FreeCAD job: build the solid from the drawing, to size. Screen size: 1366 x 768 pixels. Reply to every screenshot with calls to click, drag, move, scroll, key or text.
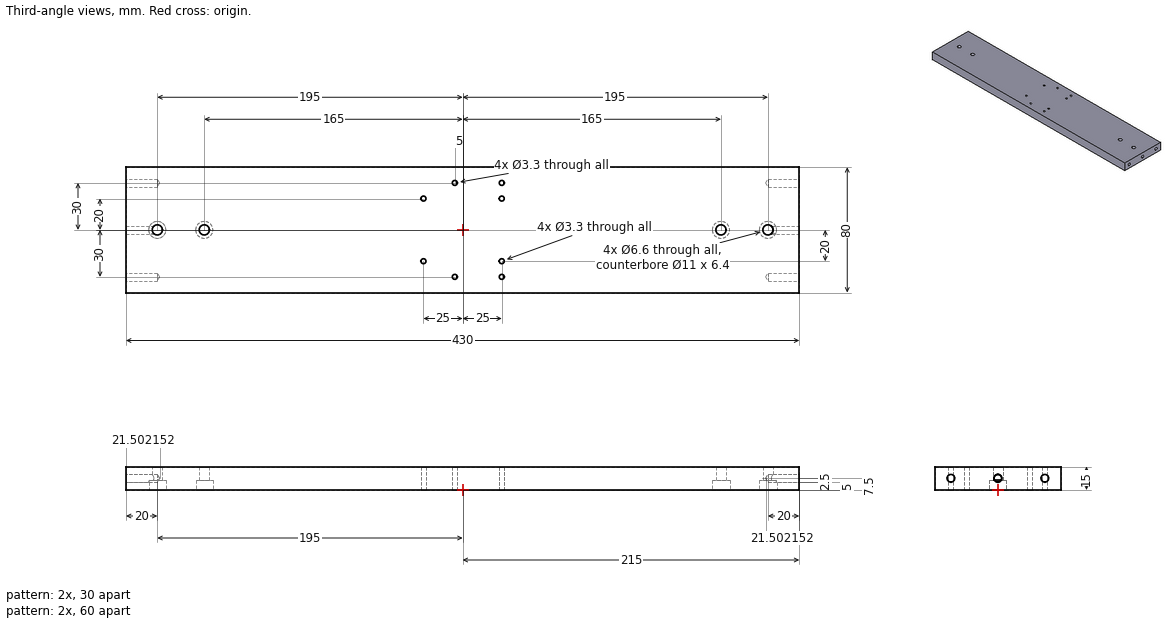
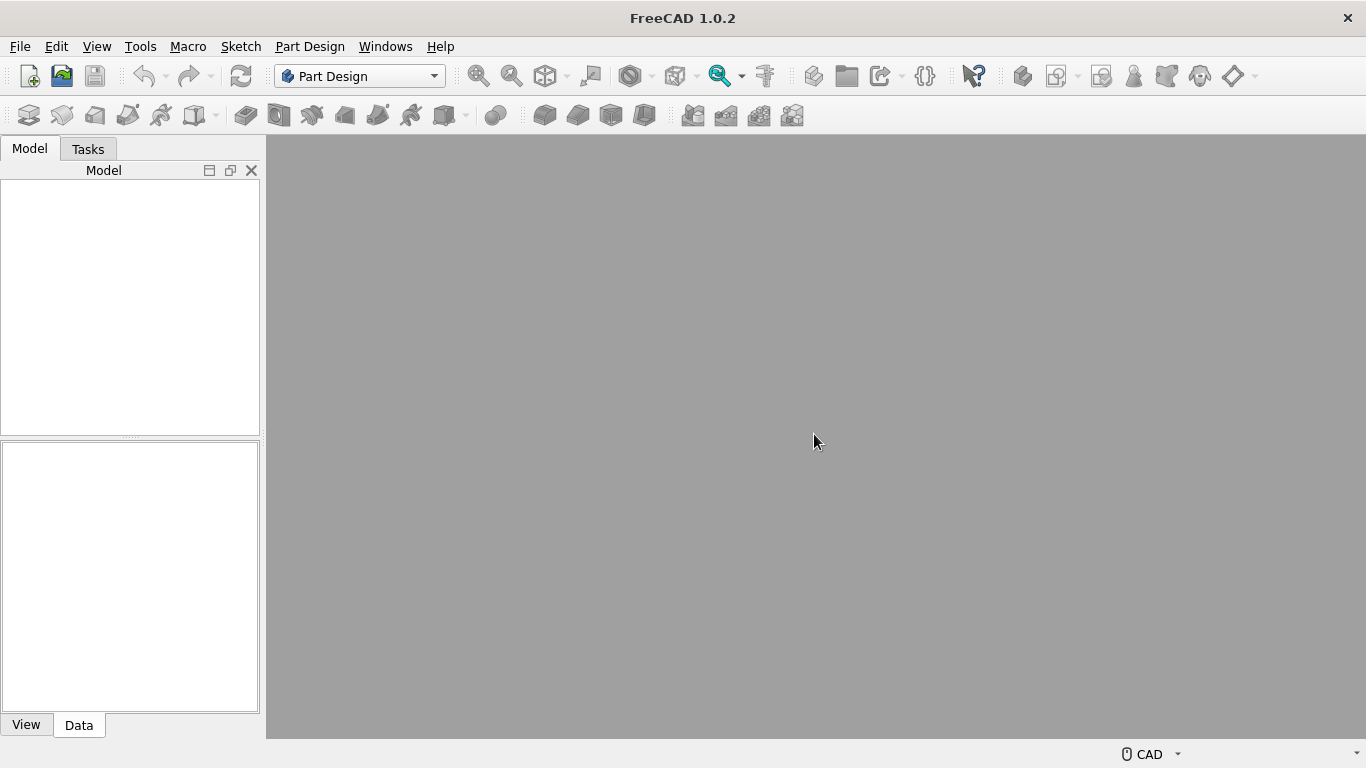
click(29, 76)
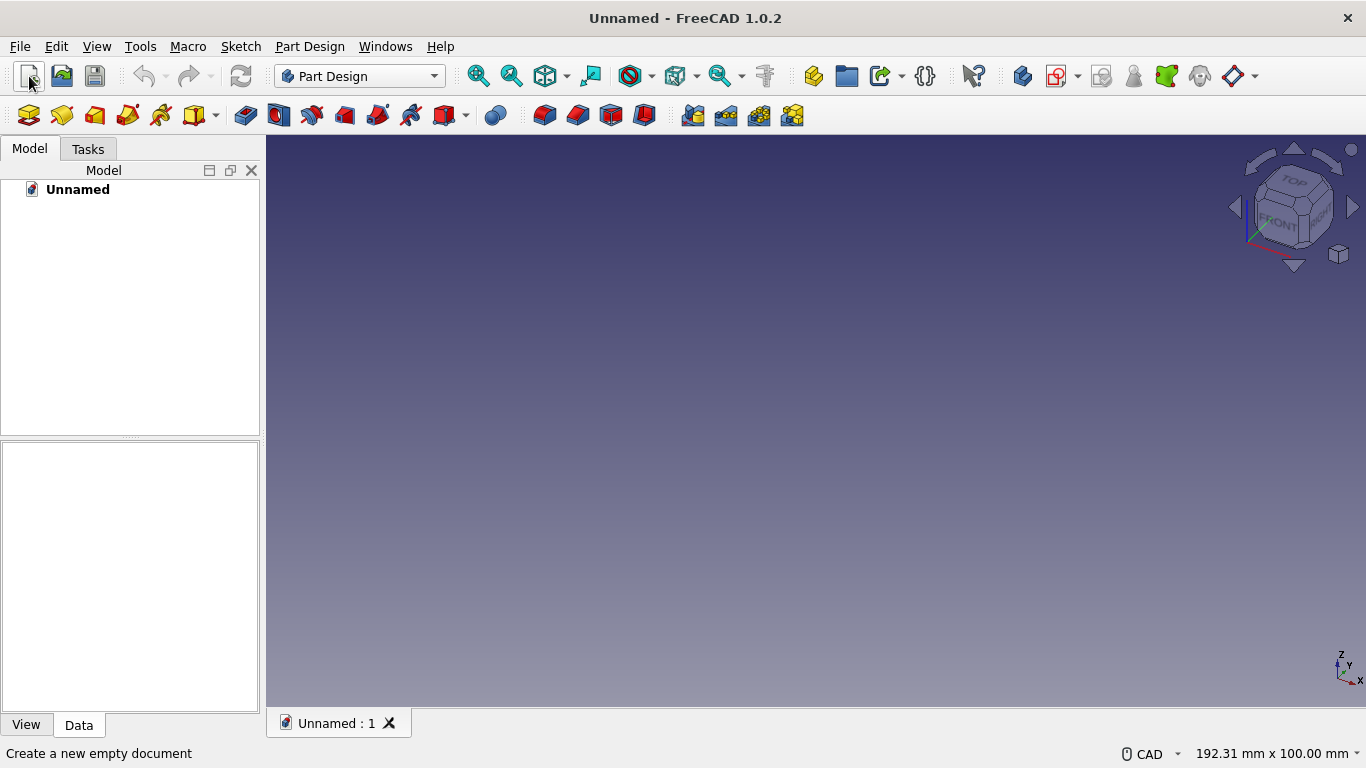
click(1056, 76)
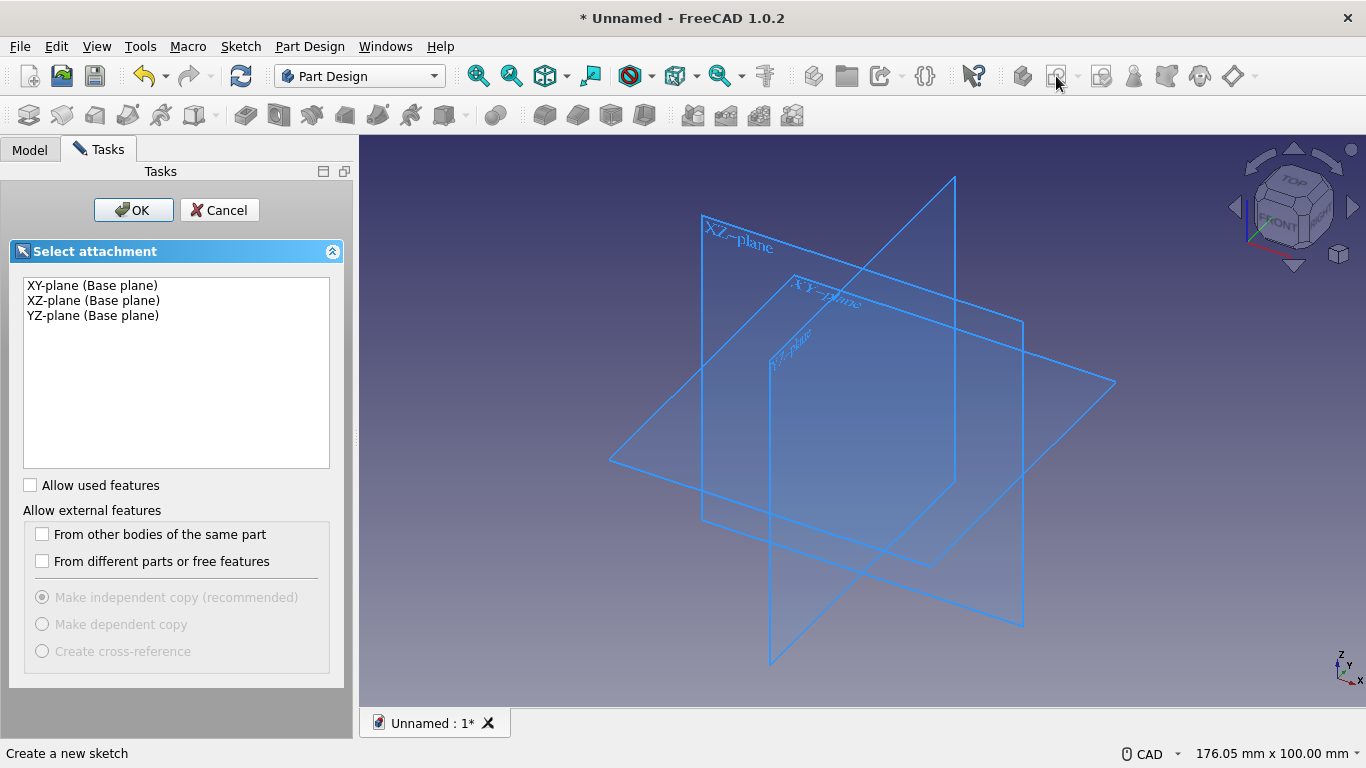
click(84, 286)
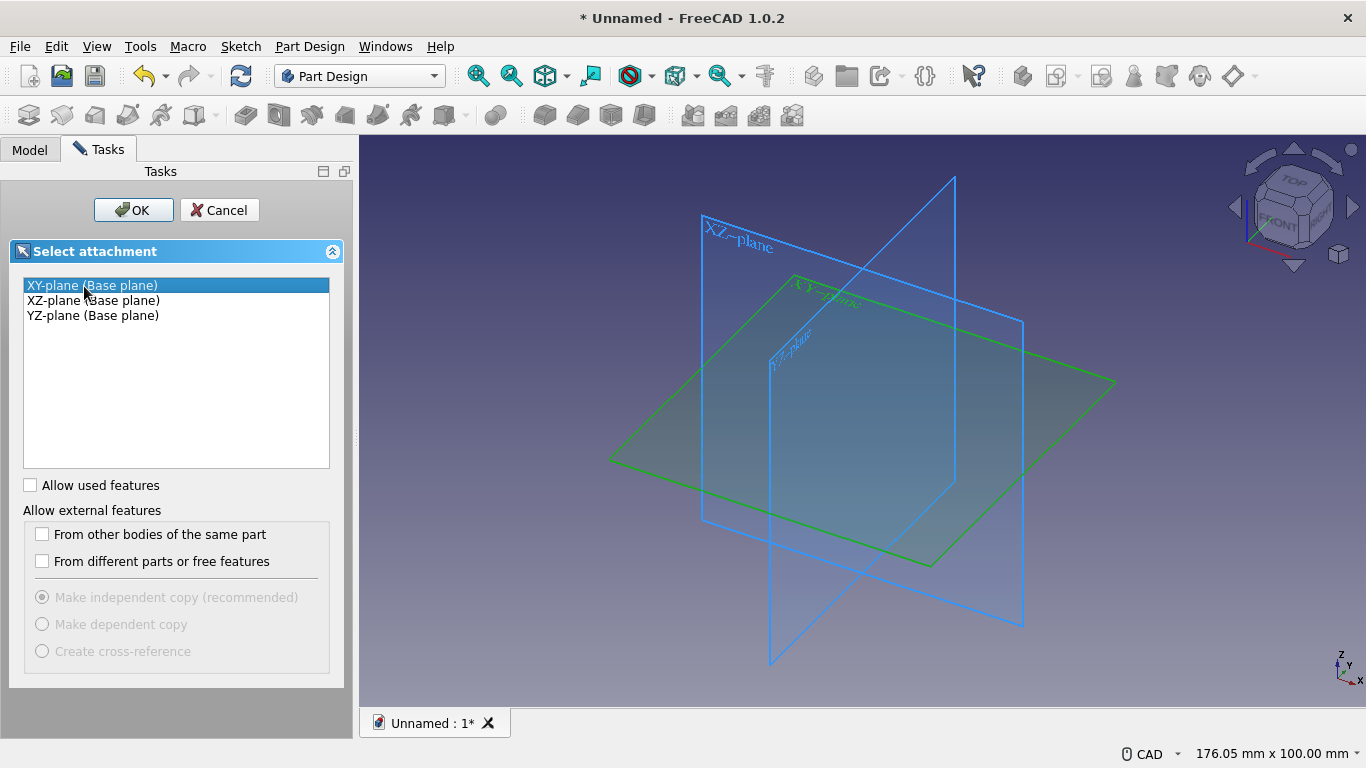
click(134, 210)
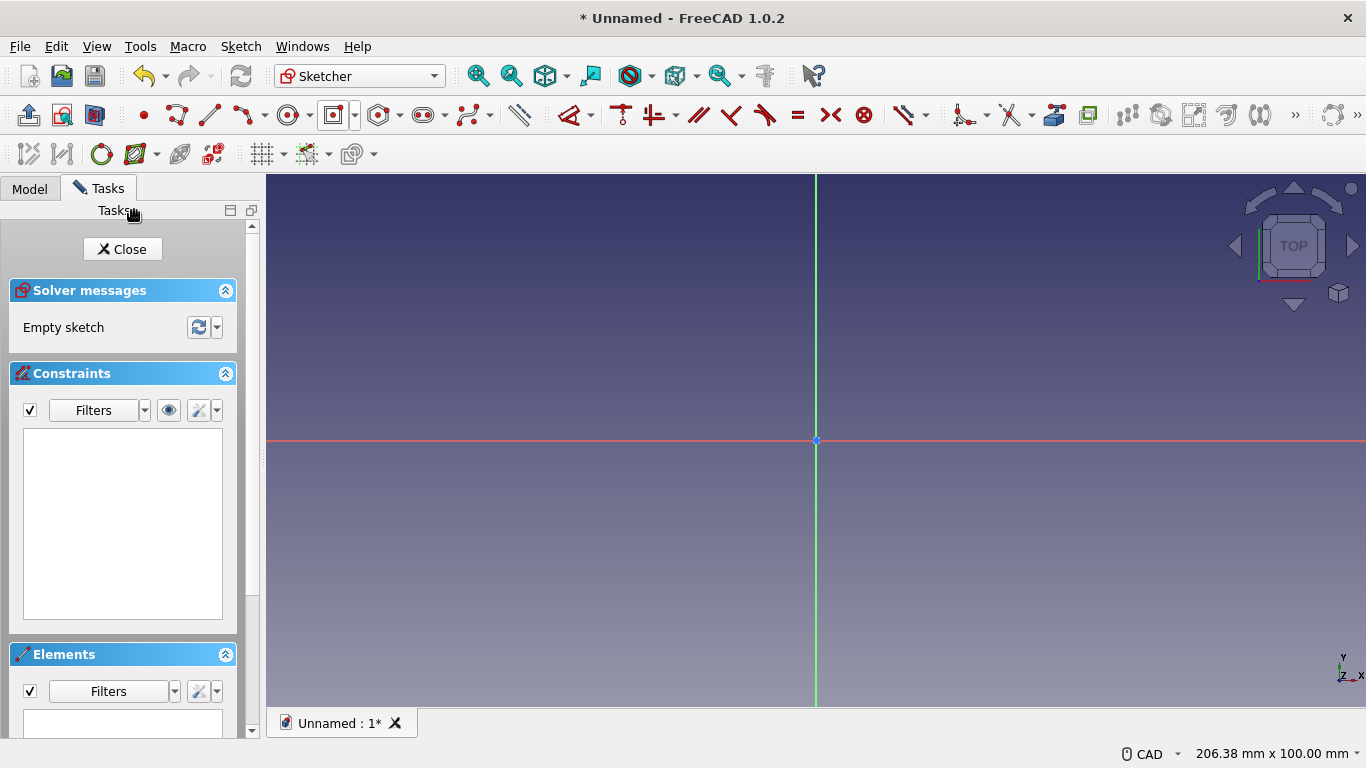
scroll(718, 440, down, 6)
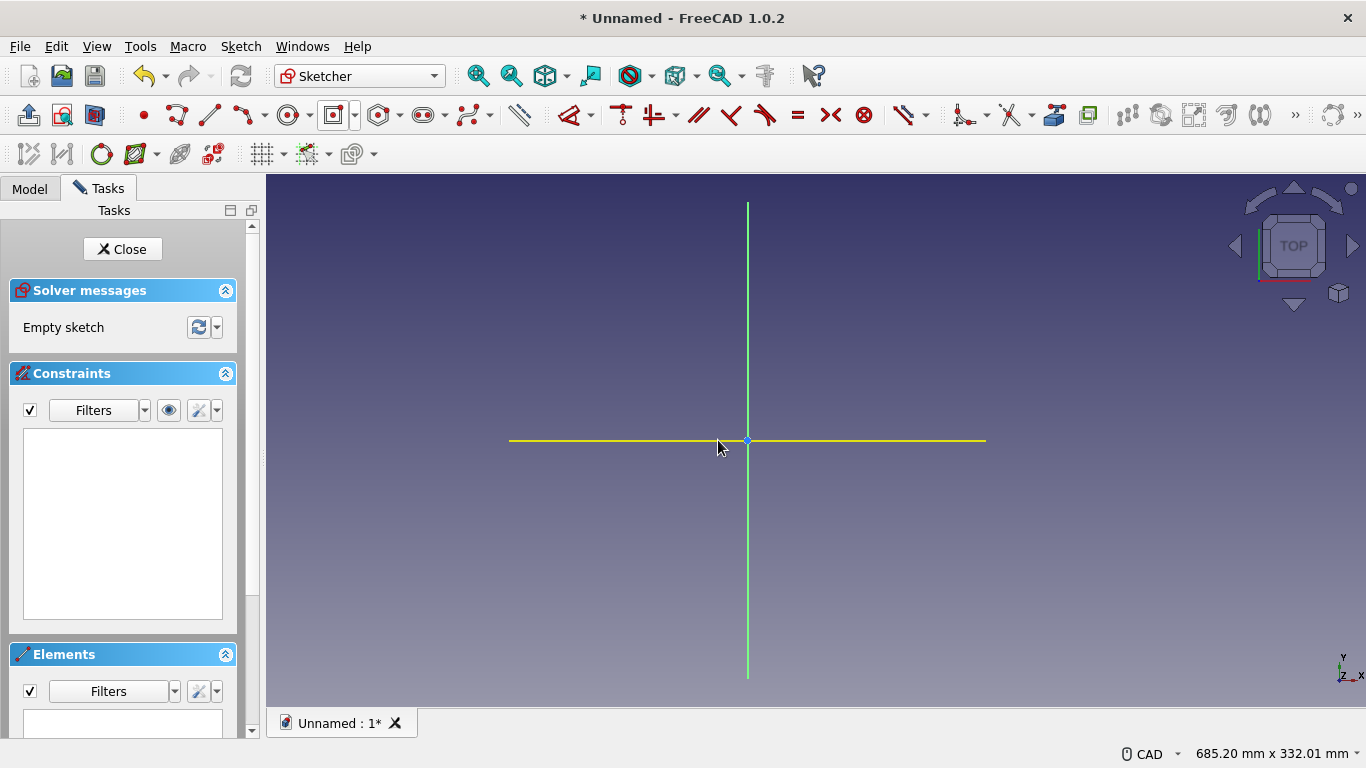
key(g)
key(v)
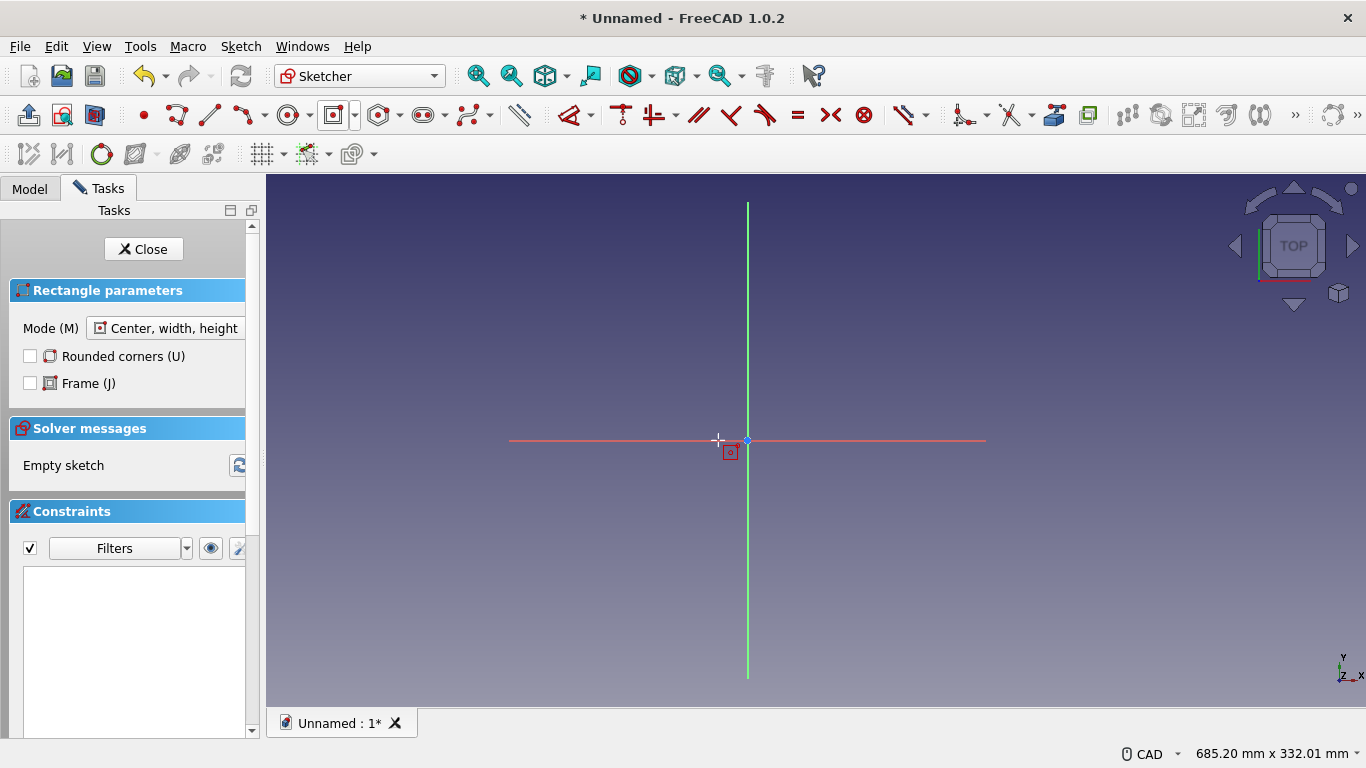
click(748, 440)
click(1093, 376)
key(Escape)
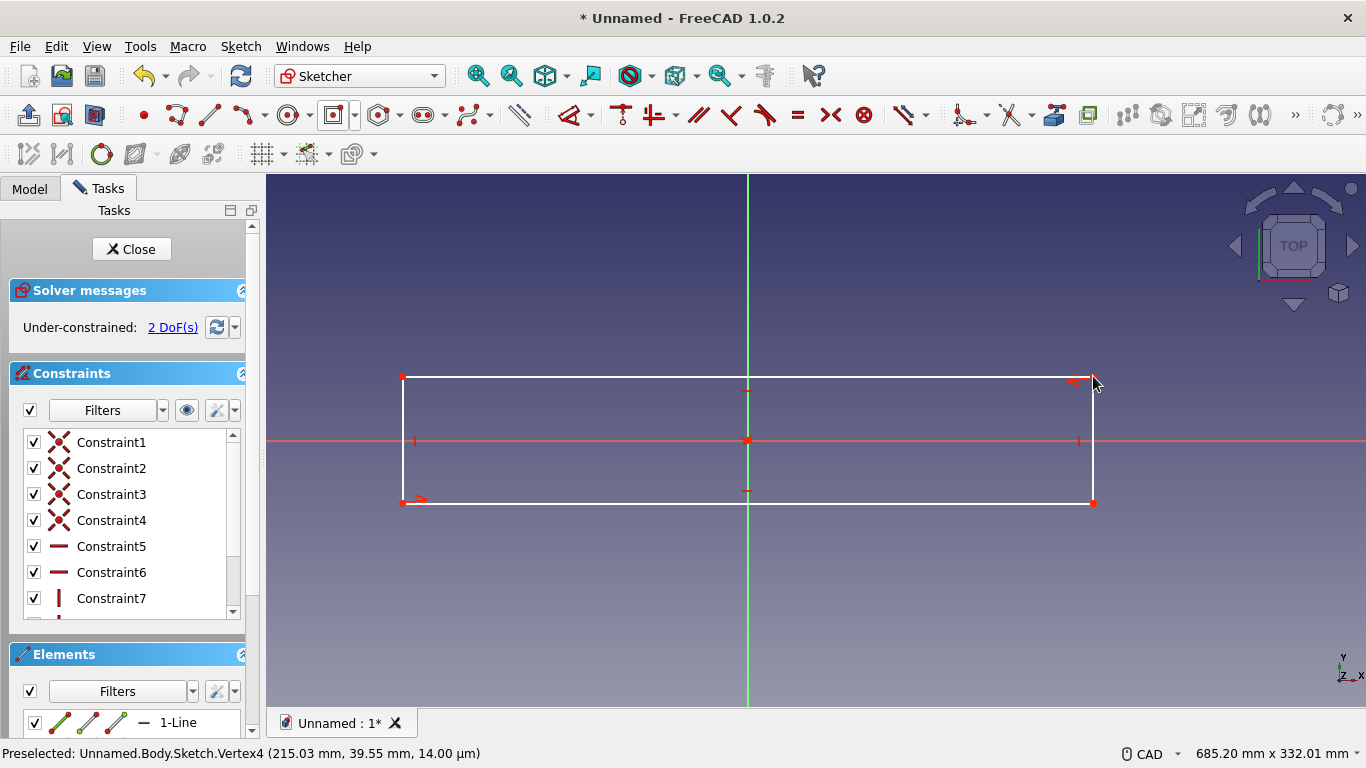
key(d)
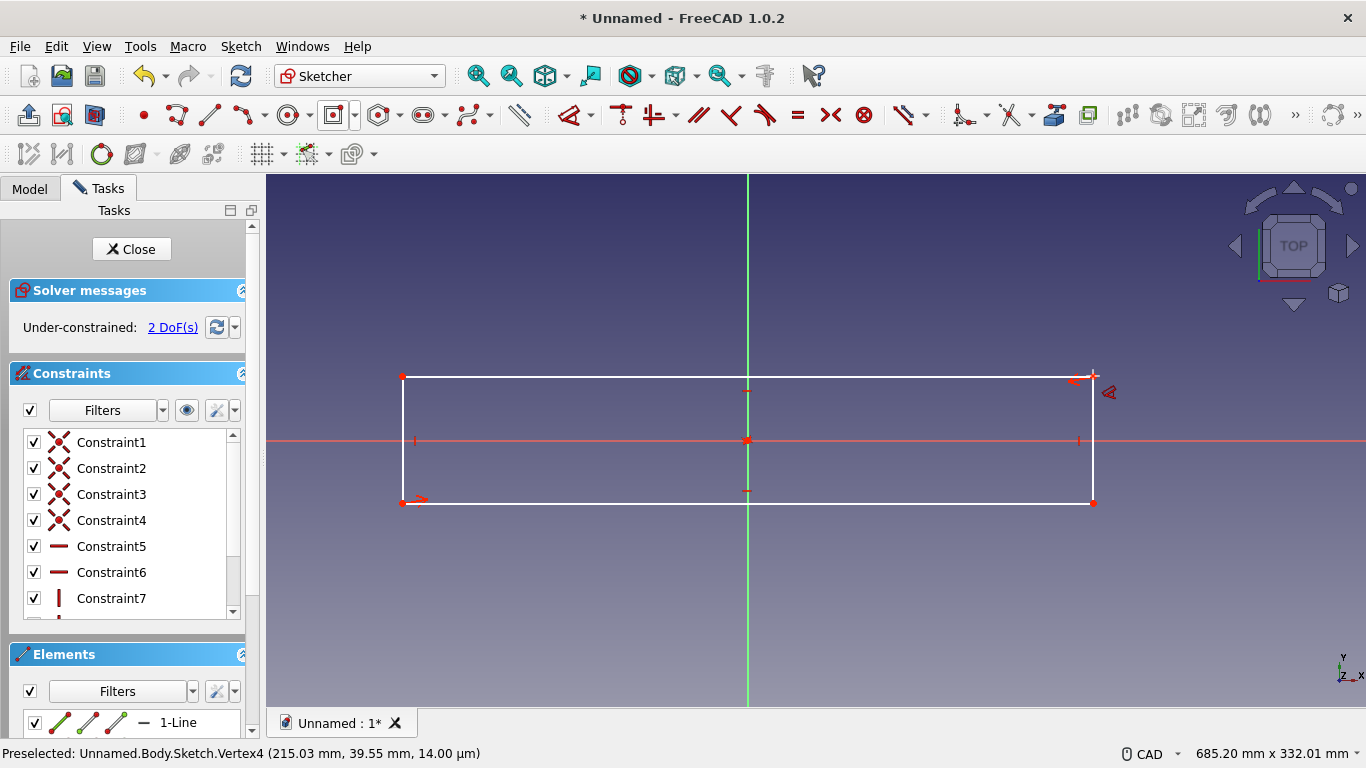
click(1093, 466)
click(1127, 411)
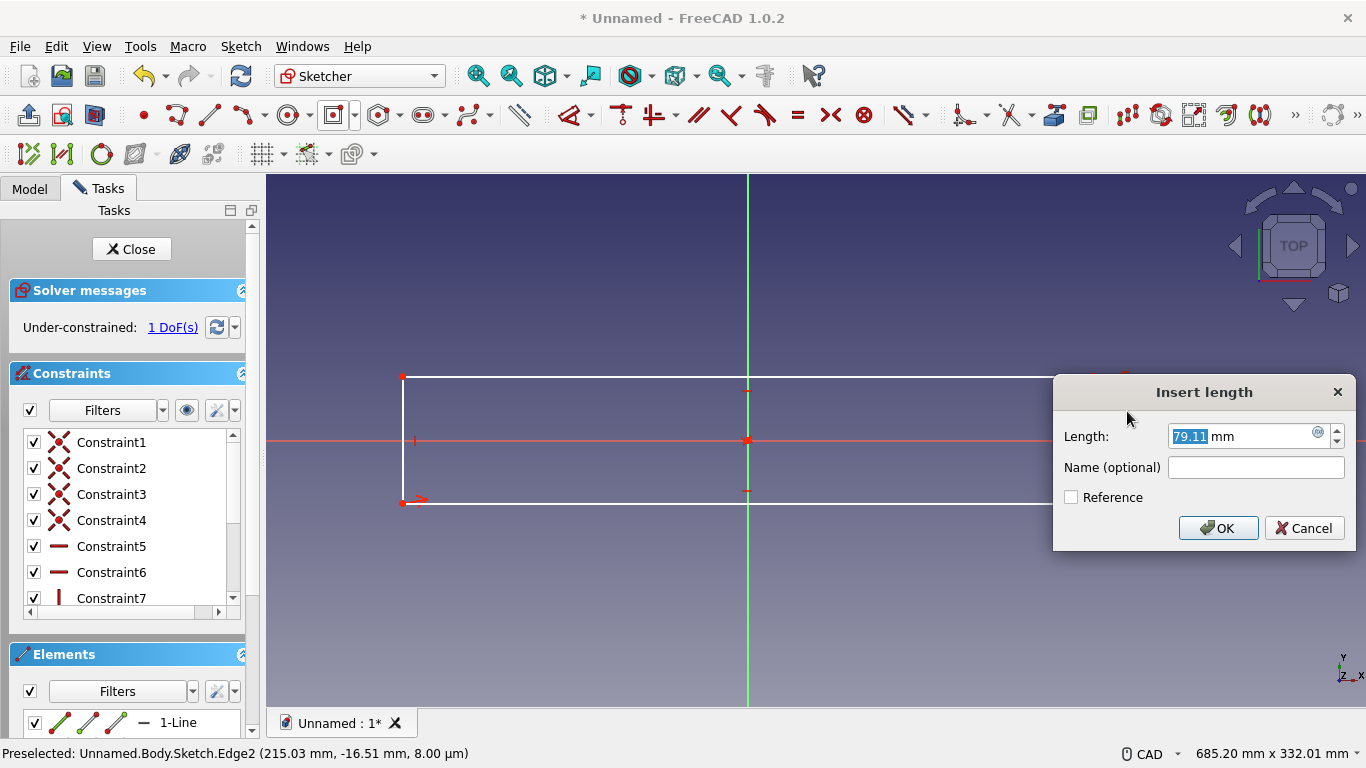
text(80)
key(Return)